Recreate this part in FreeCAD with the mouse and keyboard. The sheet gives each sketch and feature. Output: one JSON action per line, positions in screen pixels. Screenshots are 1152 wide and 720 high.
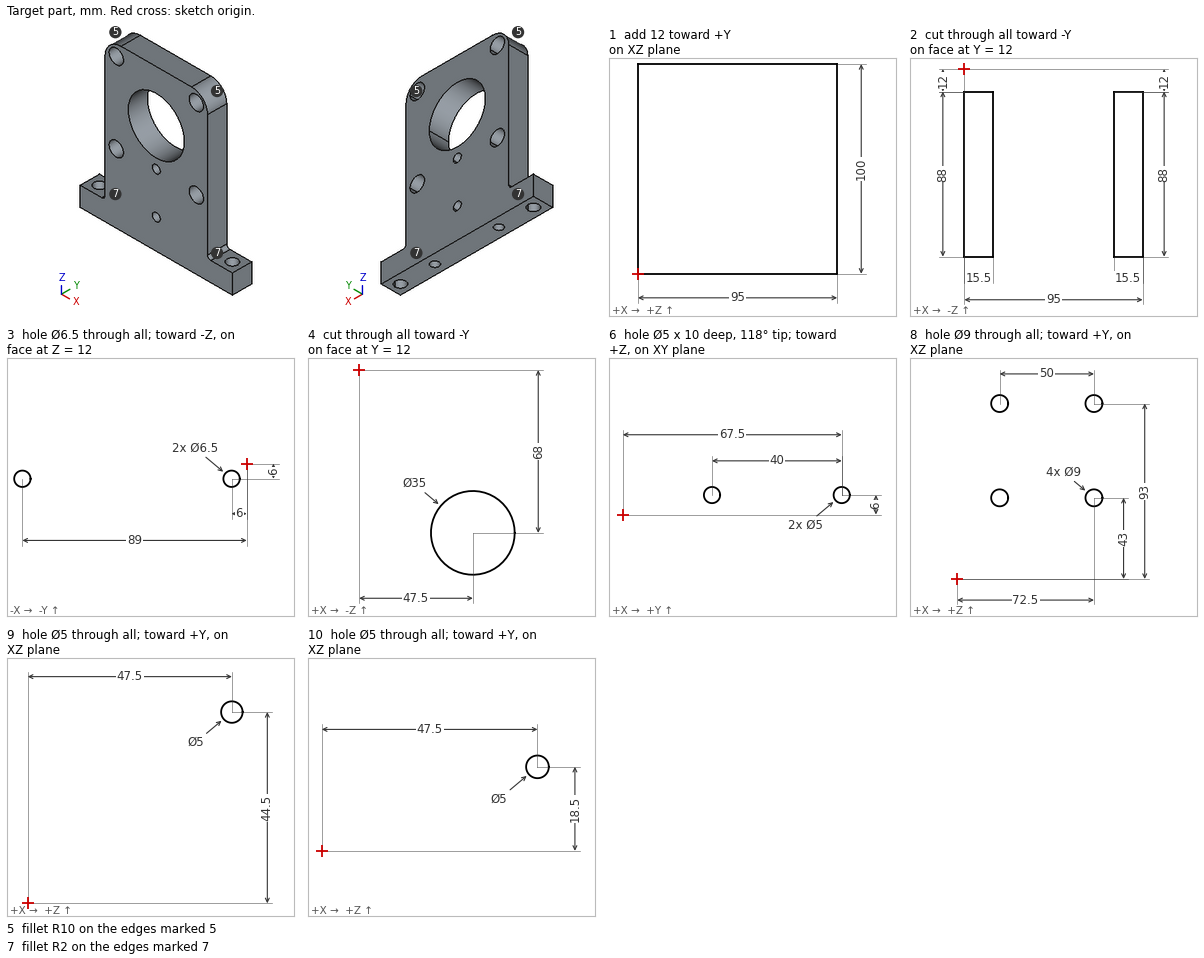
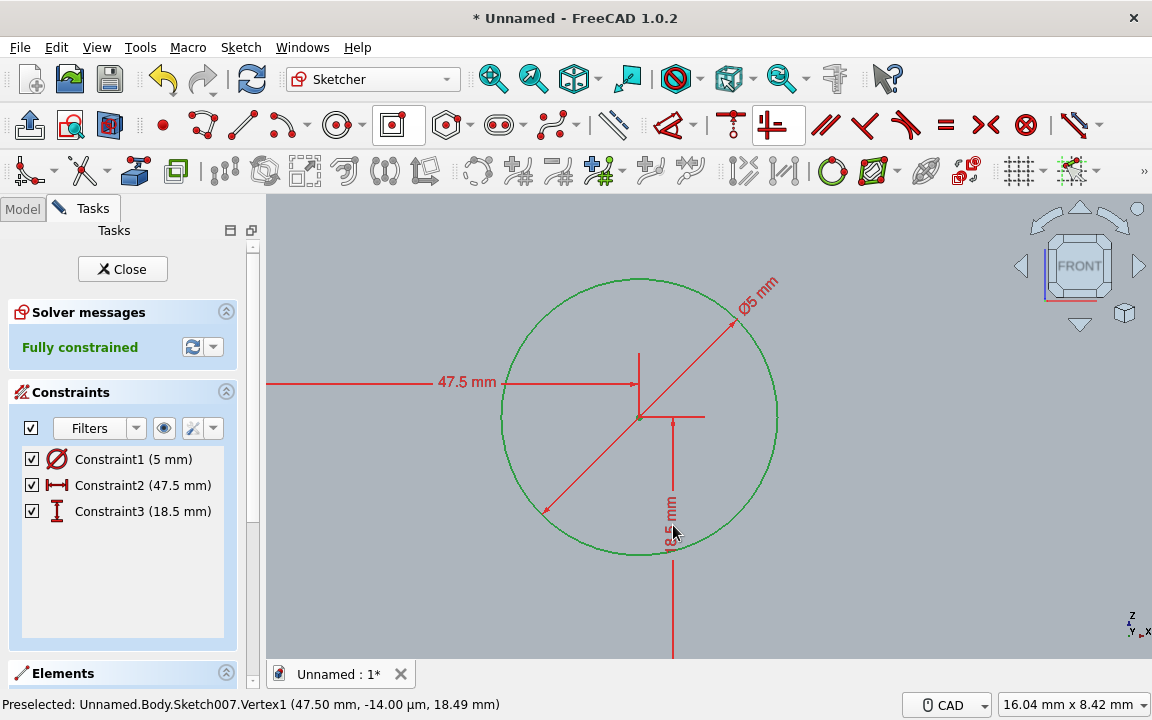
{"action": "left_click", "coordinate": [123, 269]}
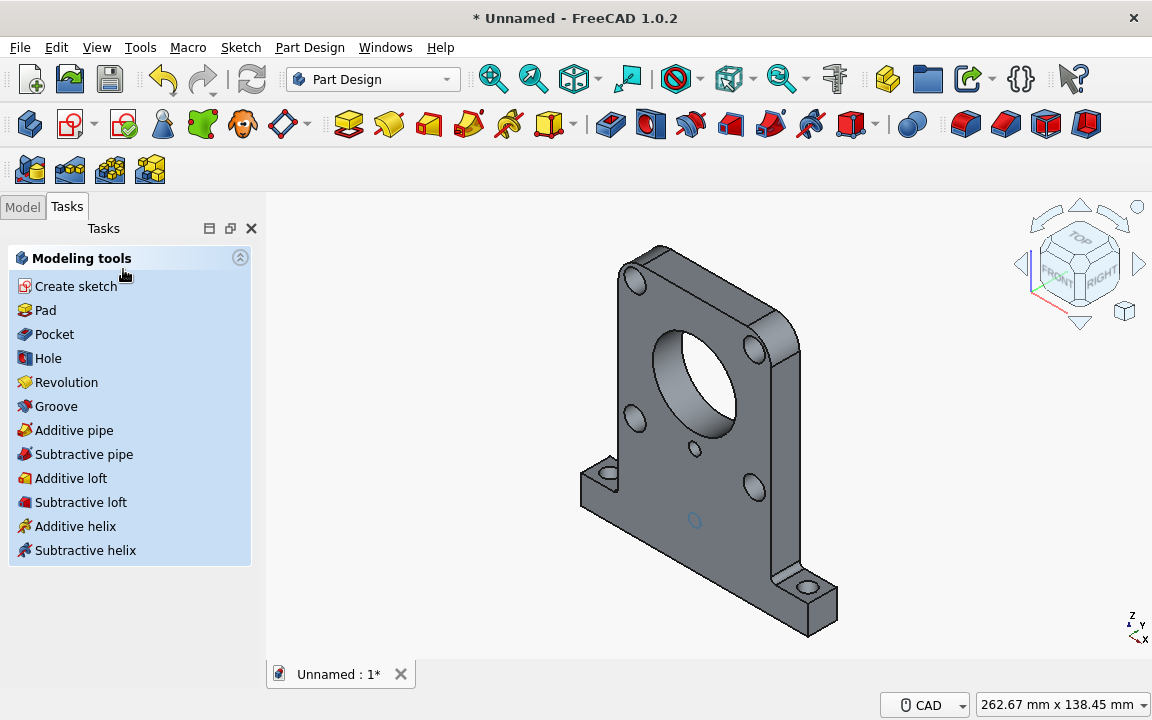
{"action": "left_click", "coordinate": [652, 124]}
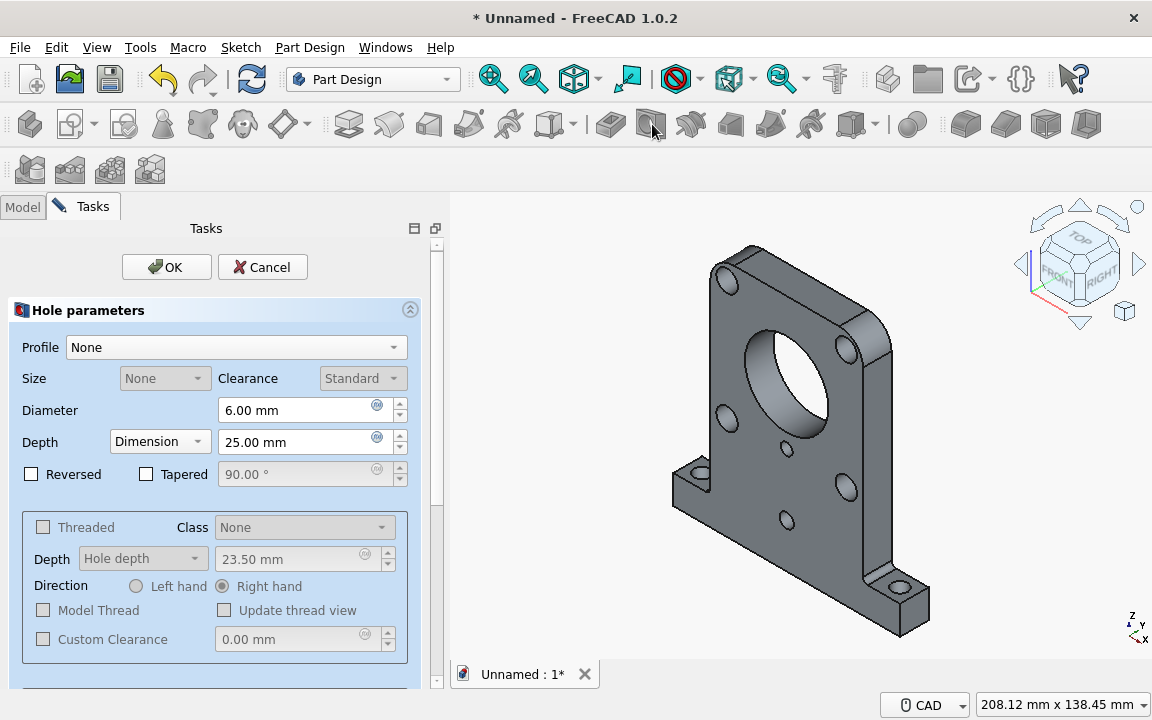
{"action": "triple_click", "coordinate": [305, 410]}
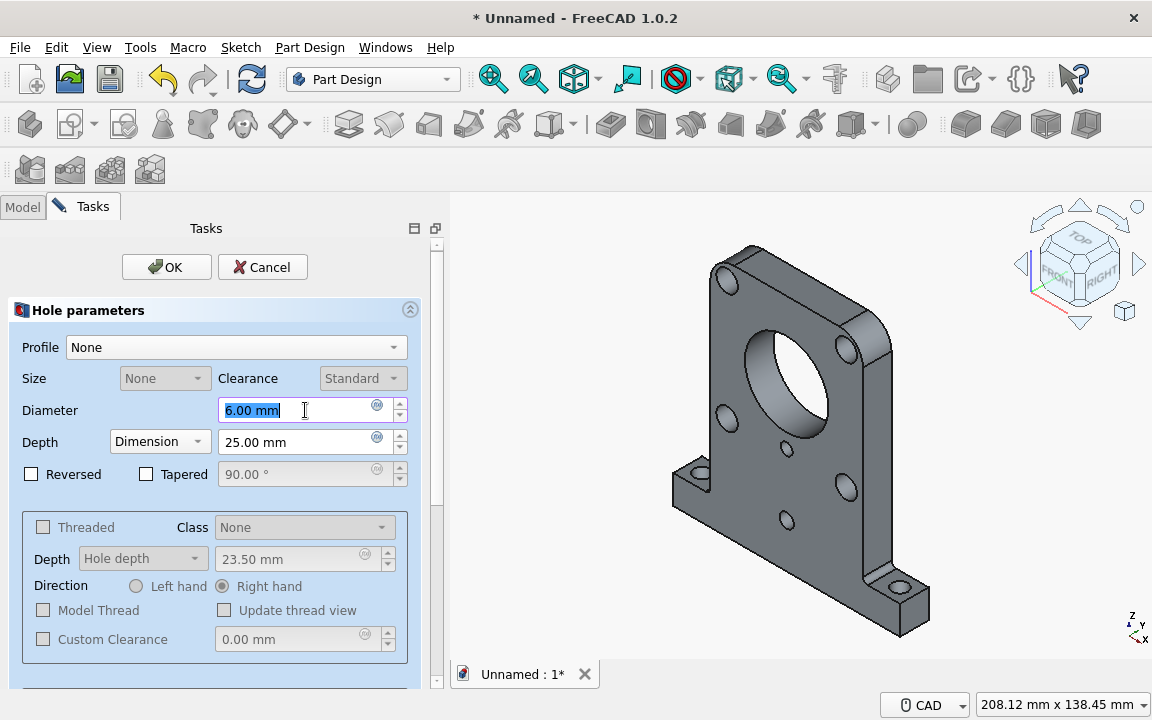
{"action": "type", "text": "5"}
{"action": "key", "text": "Tab"}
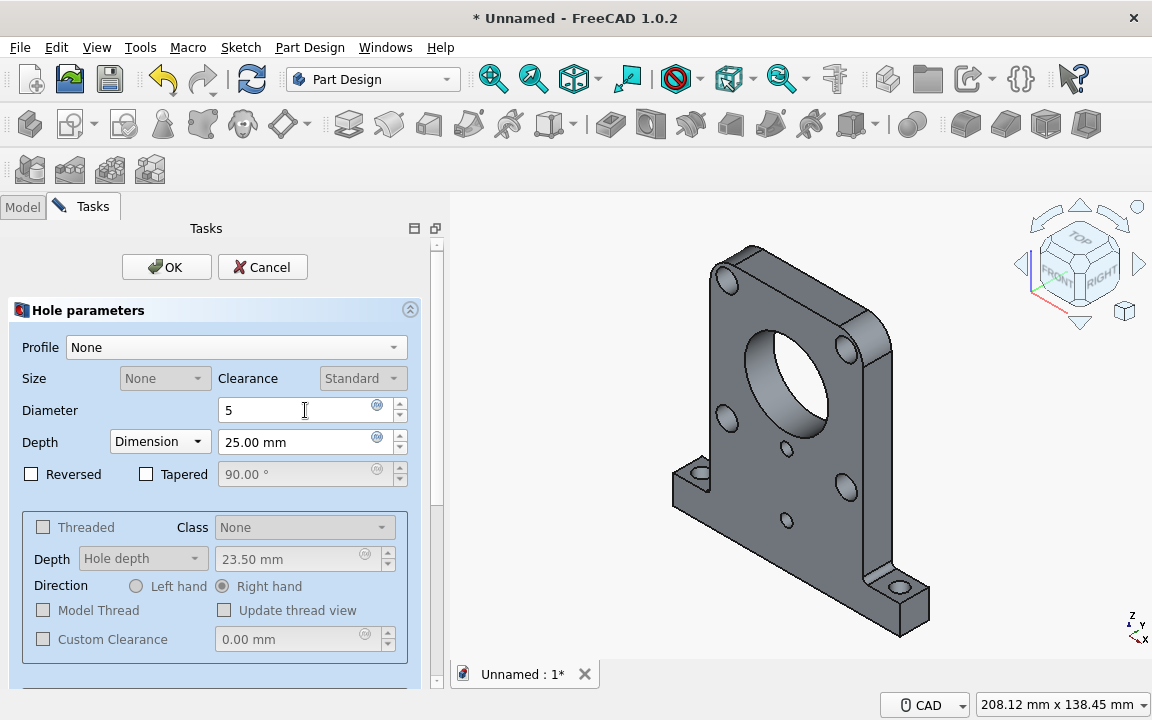
{"action": "left_click", "coordinate": [161, 442]}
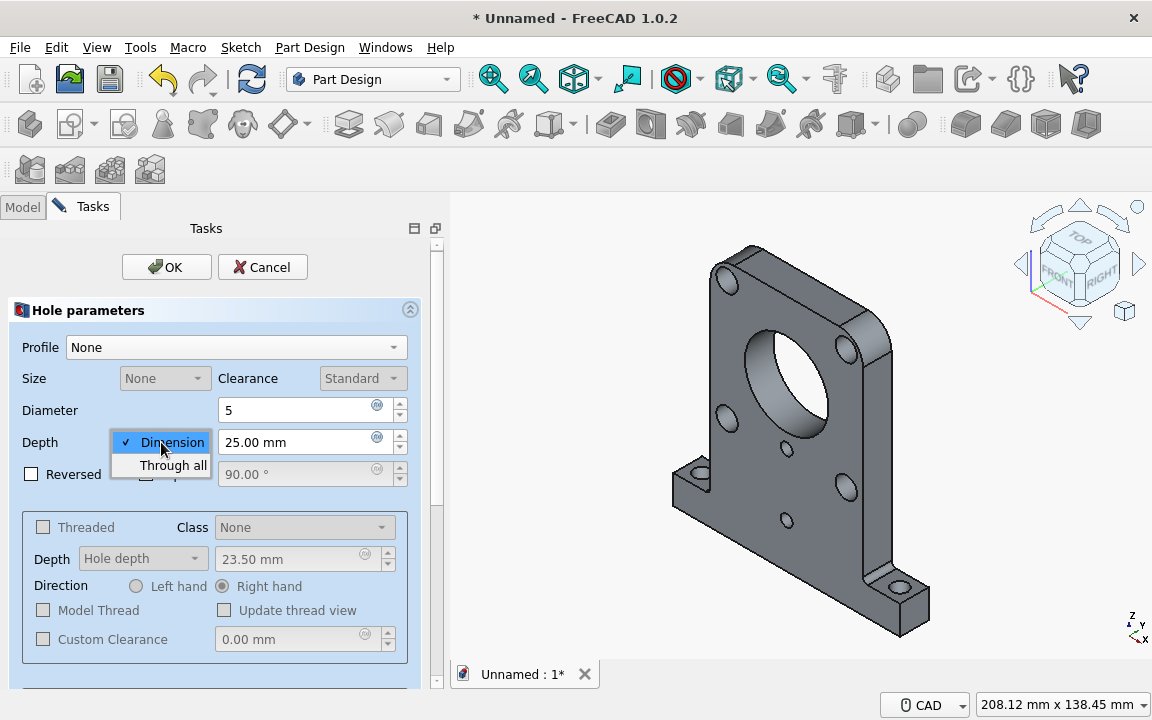
{"action": "left_click", "coordinate": [160, 466]}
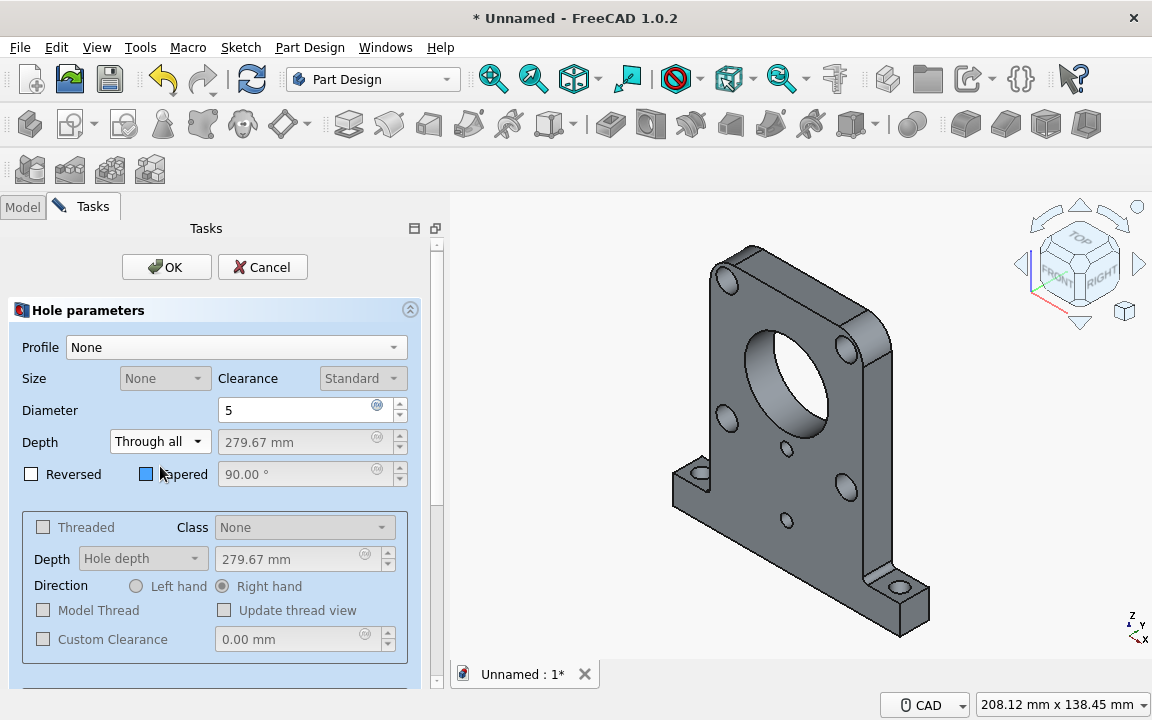
{"action": "left_click", "coordinate": [167, 267]}